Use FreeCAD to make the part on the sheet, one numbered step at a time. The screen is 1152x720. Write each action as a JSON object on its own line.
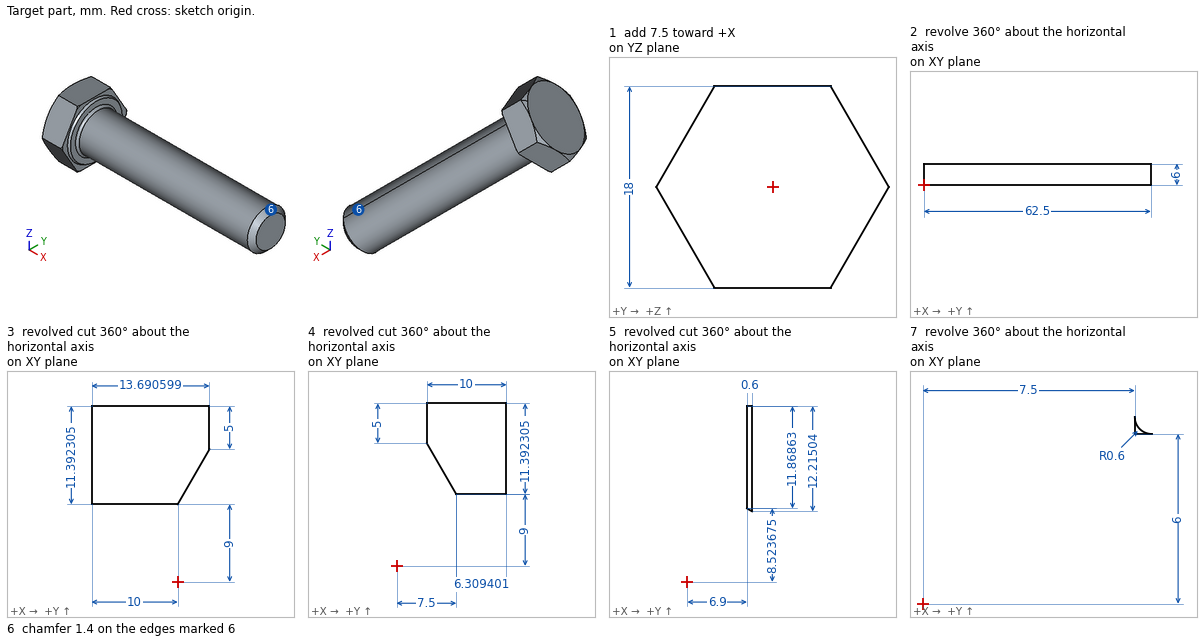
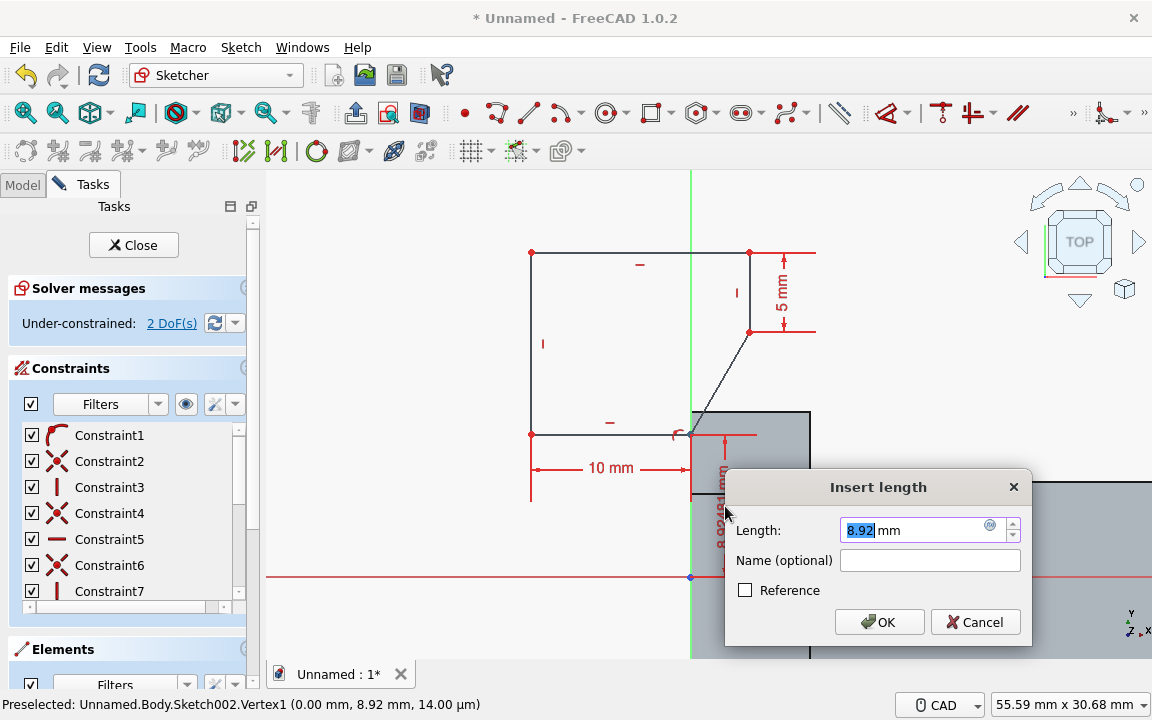
{"action": "type", "text": "9"}
{"action": "key", "text": "Return"}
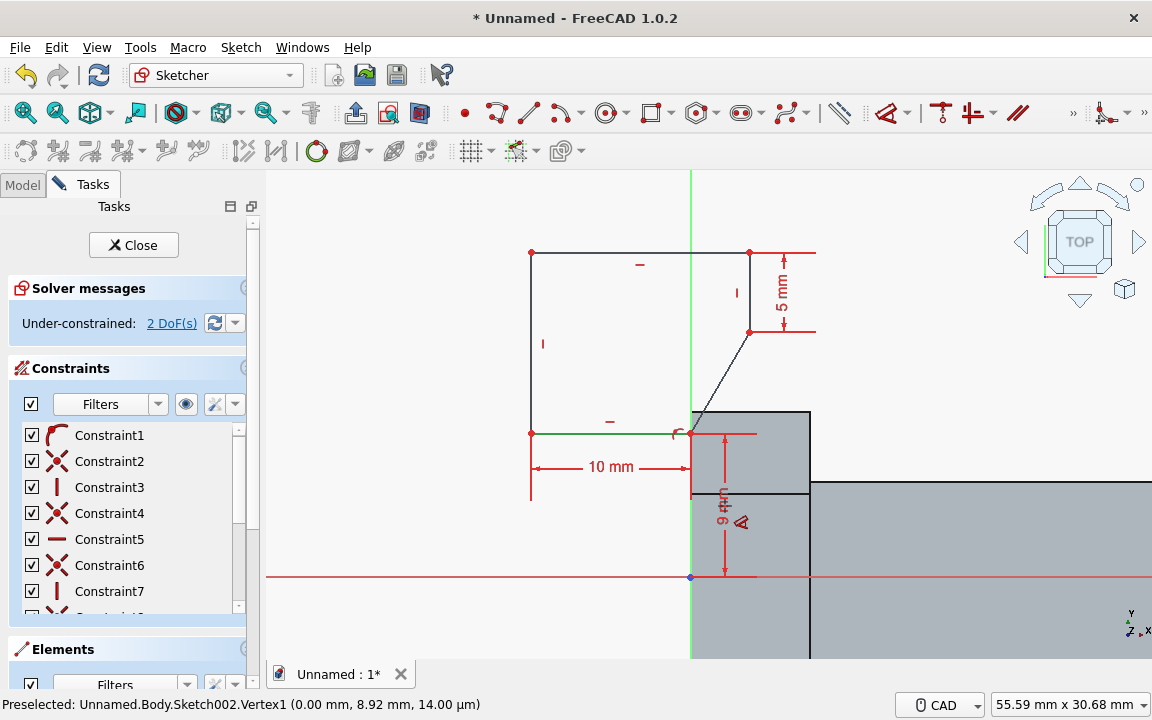
{"action": "left_click", "coordinate": [597, 253]}
{"action": "left_click", "coordinate": [640, 219]}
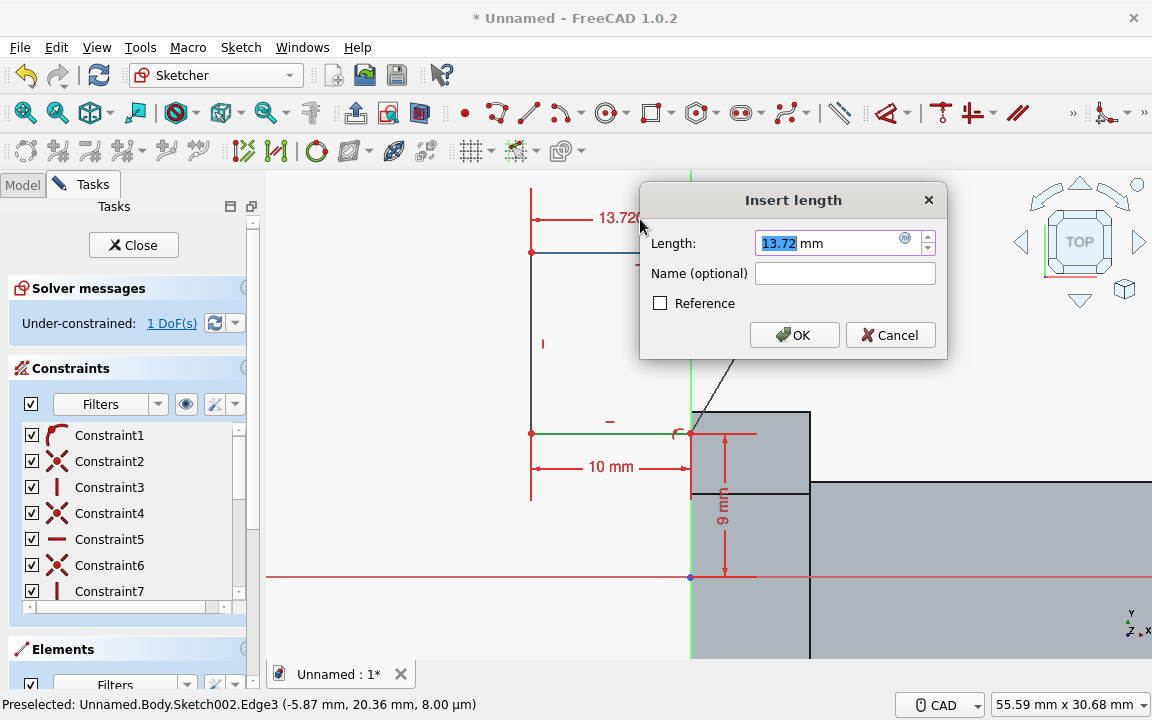
{"action": "type", "text": "13.690599"}
{"action": "key", "text": "Return"}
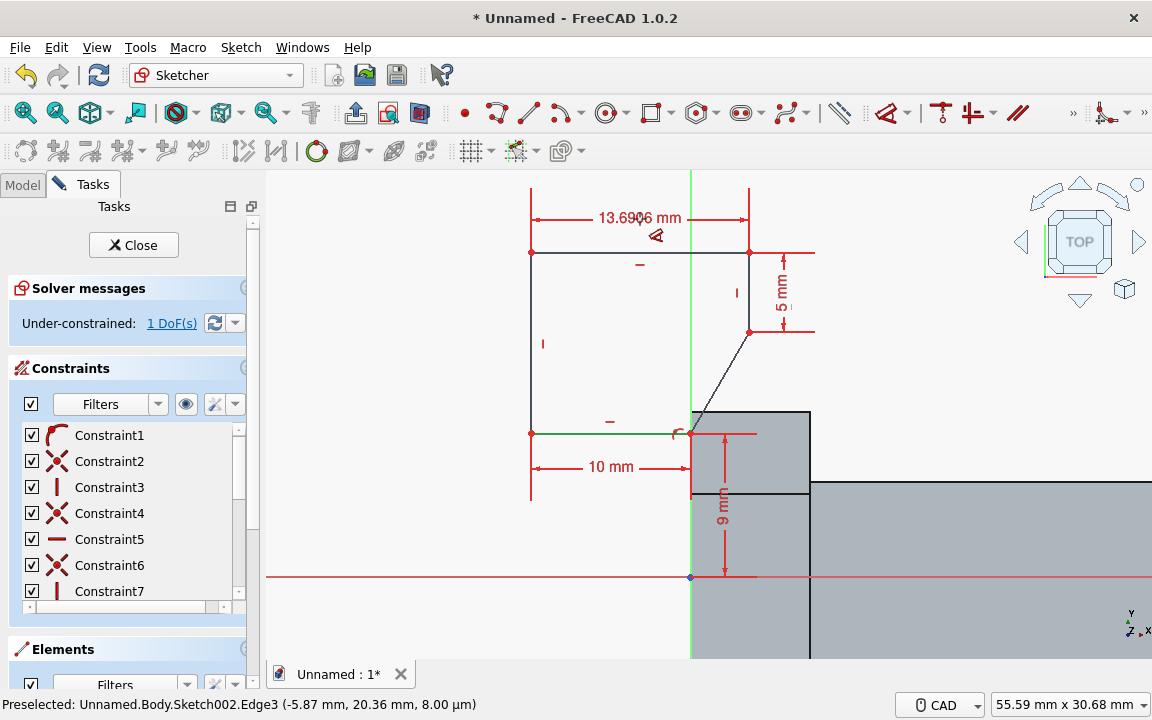
{"action": "left_click", "coordinate": [531, 307]}
{"action": "left_click", "coordinate": [497, 343]}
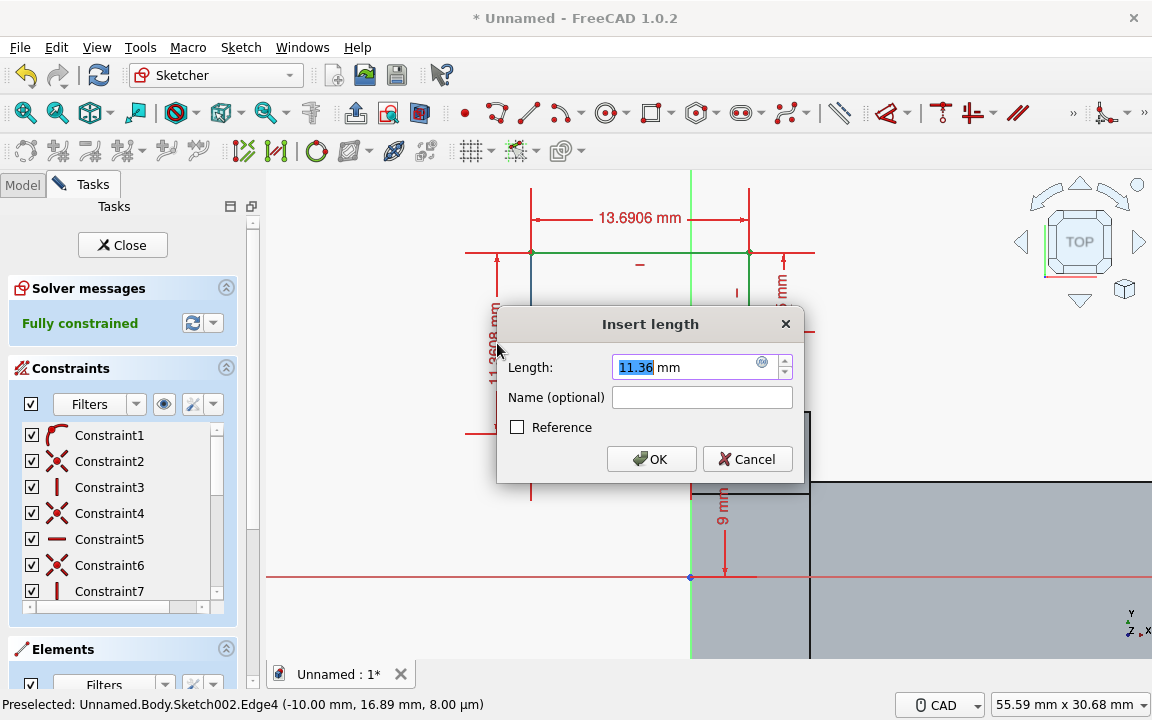
{"action": "type", "text": "11.392305"}
{"action": "key", "text": "Return"}
{"action": "key", "text": "Escape"}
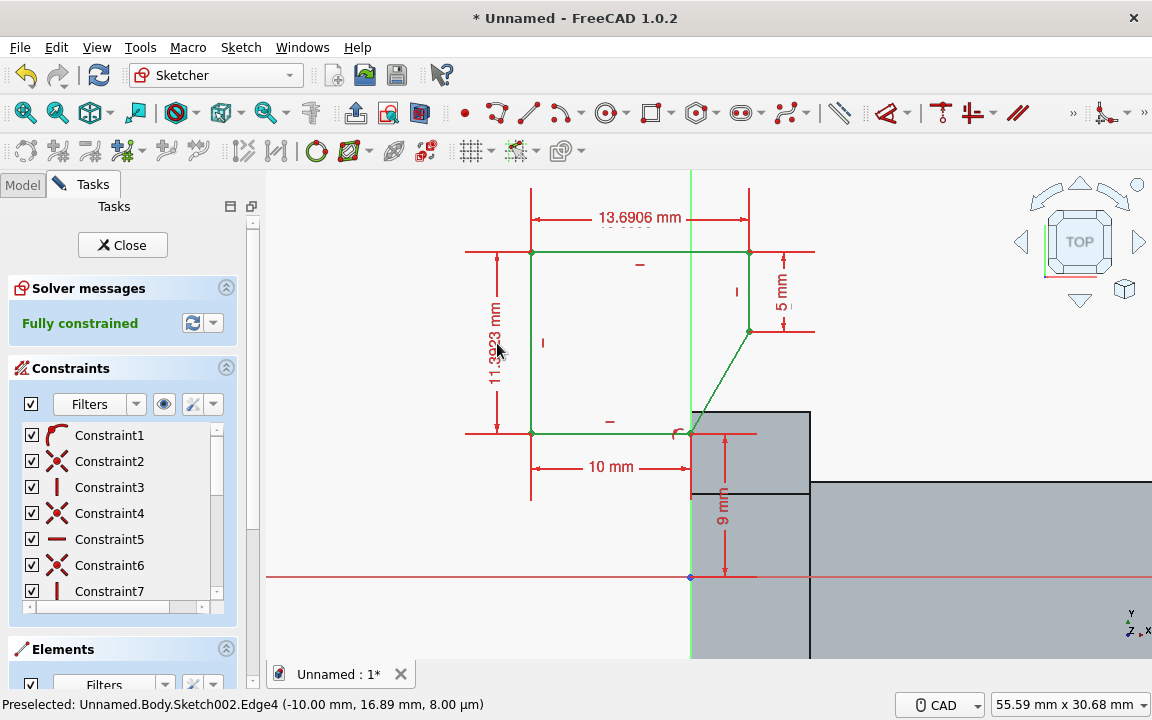
{"action": "left_click", "coordinate": [123, 245]}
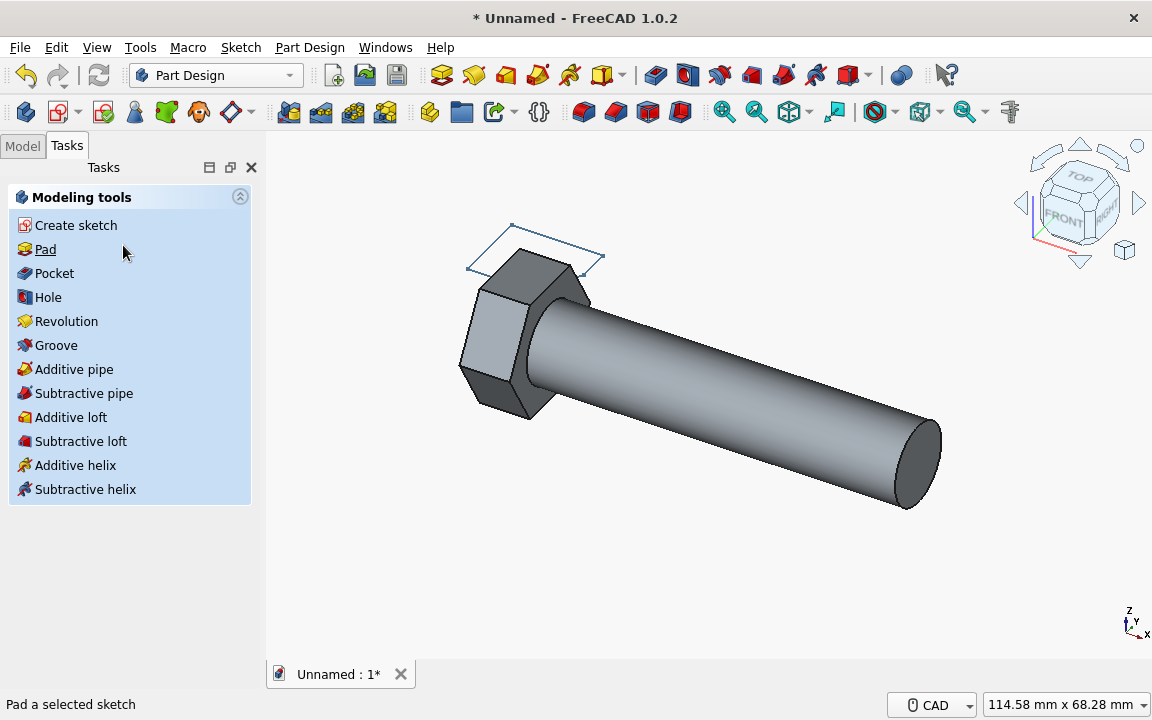
{"action": "left_click", "coordinate": [720, 76]}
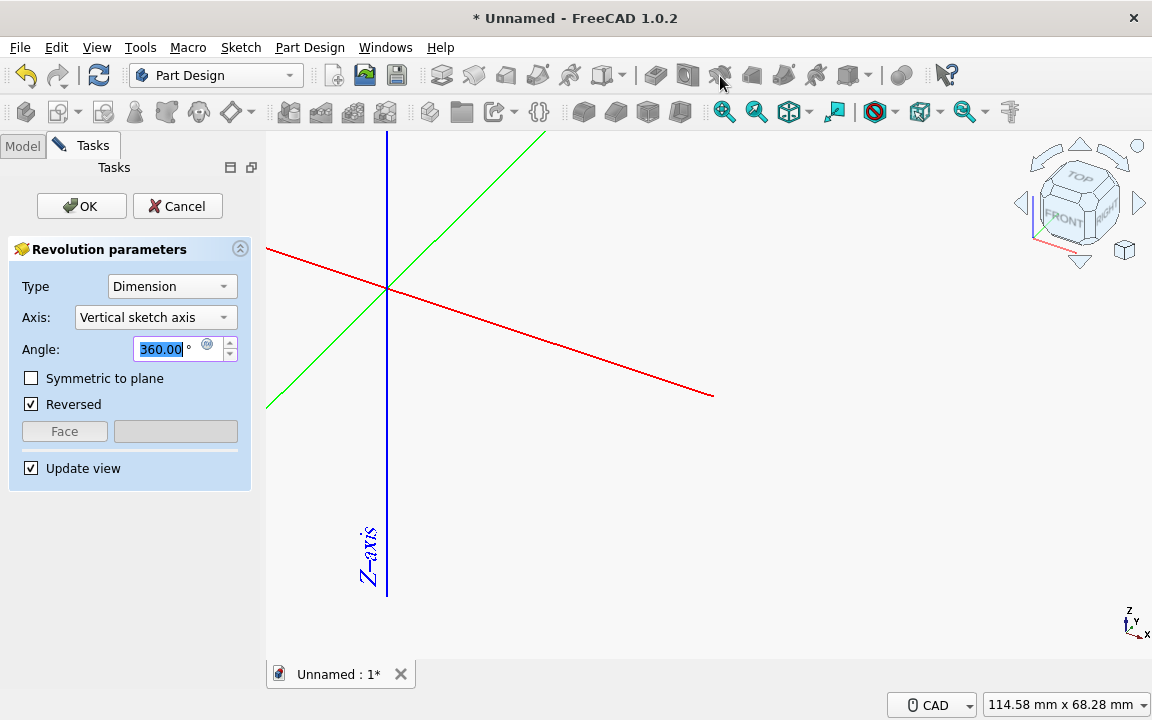
{"action": "left_click", "coordinate": [156, 318]}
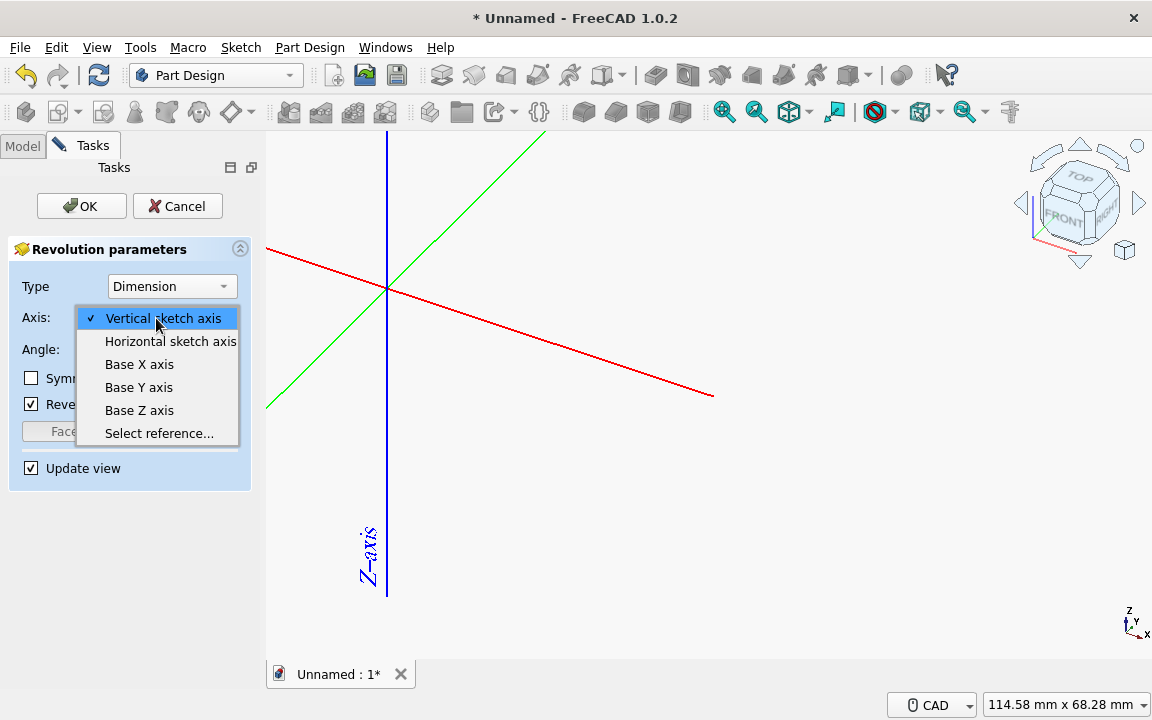
{"action": "left_click", "coordinate": [156, 342]}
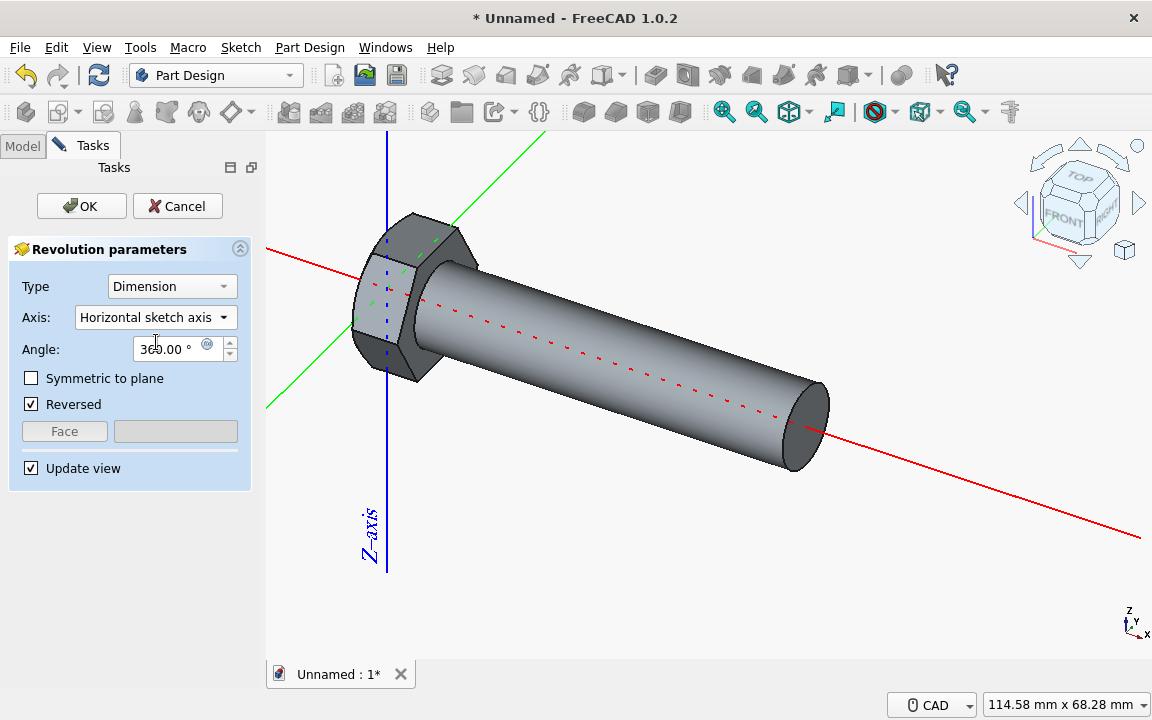
{"action": "left_click", "coordinate": [82, 206]}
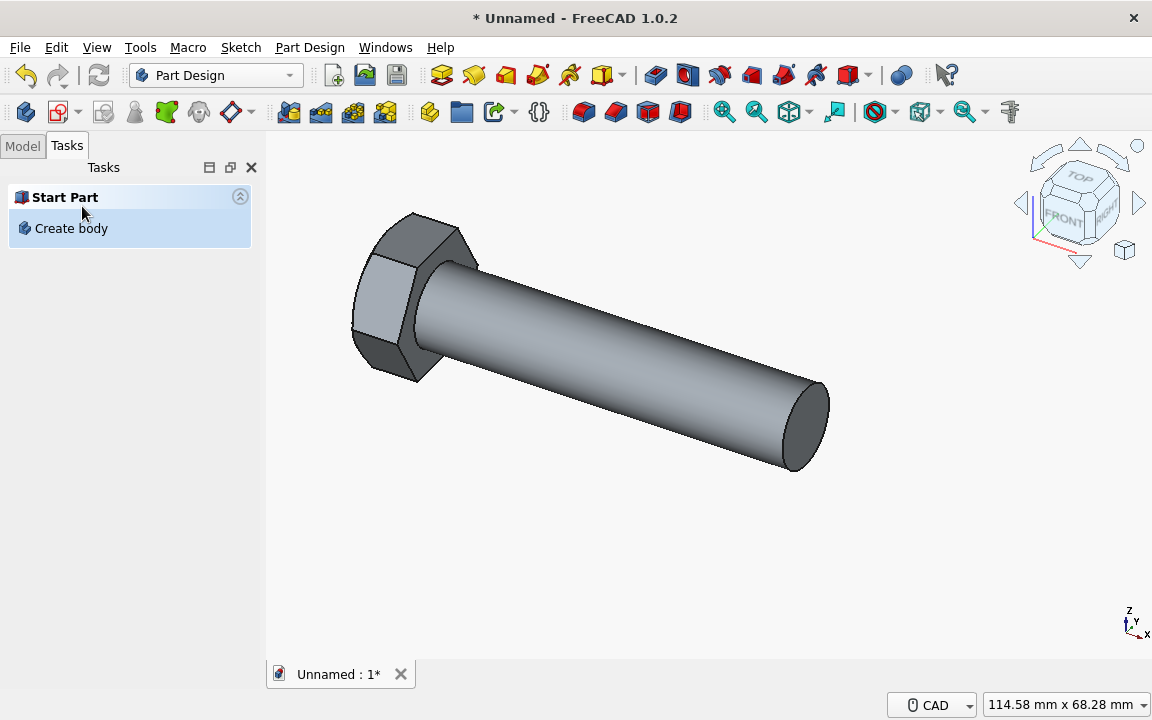
{"action": "left_click", "coordinate": [58, 112]}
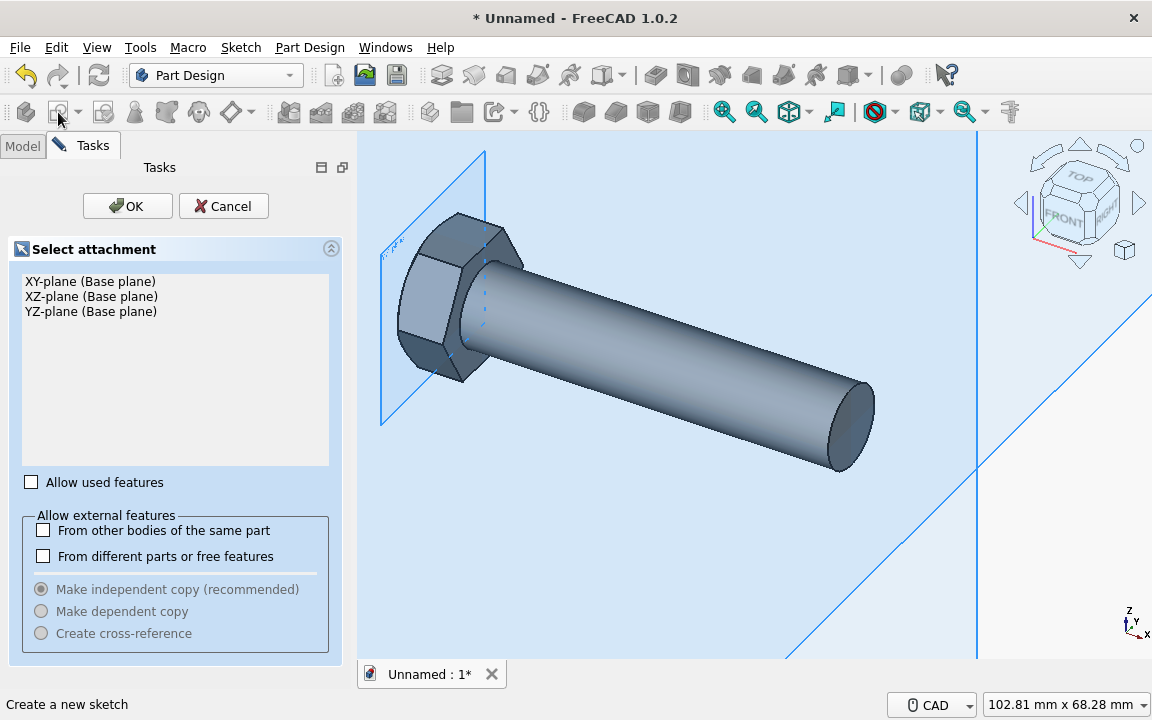
{"action": "left_click", "coordinate": [82, 282]}